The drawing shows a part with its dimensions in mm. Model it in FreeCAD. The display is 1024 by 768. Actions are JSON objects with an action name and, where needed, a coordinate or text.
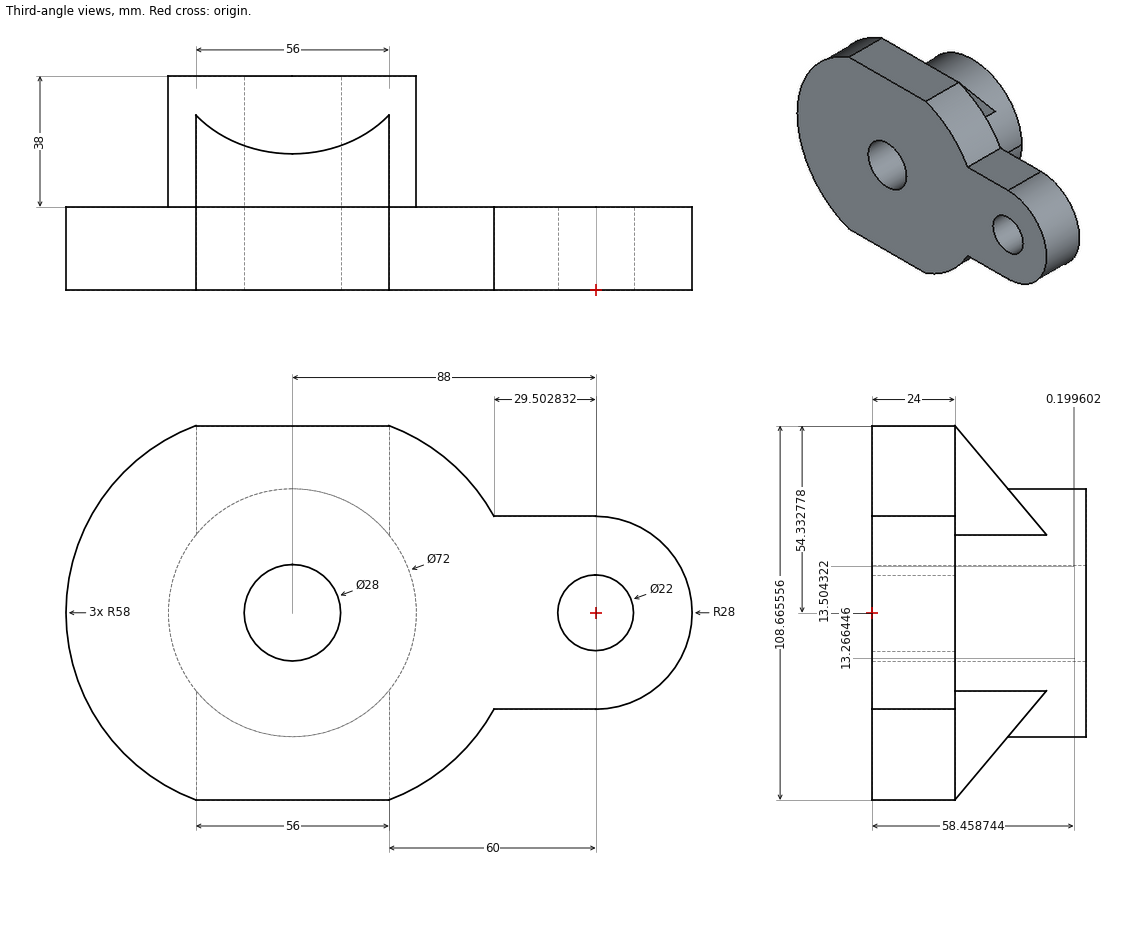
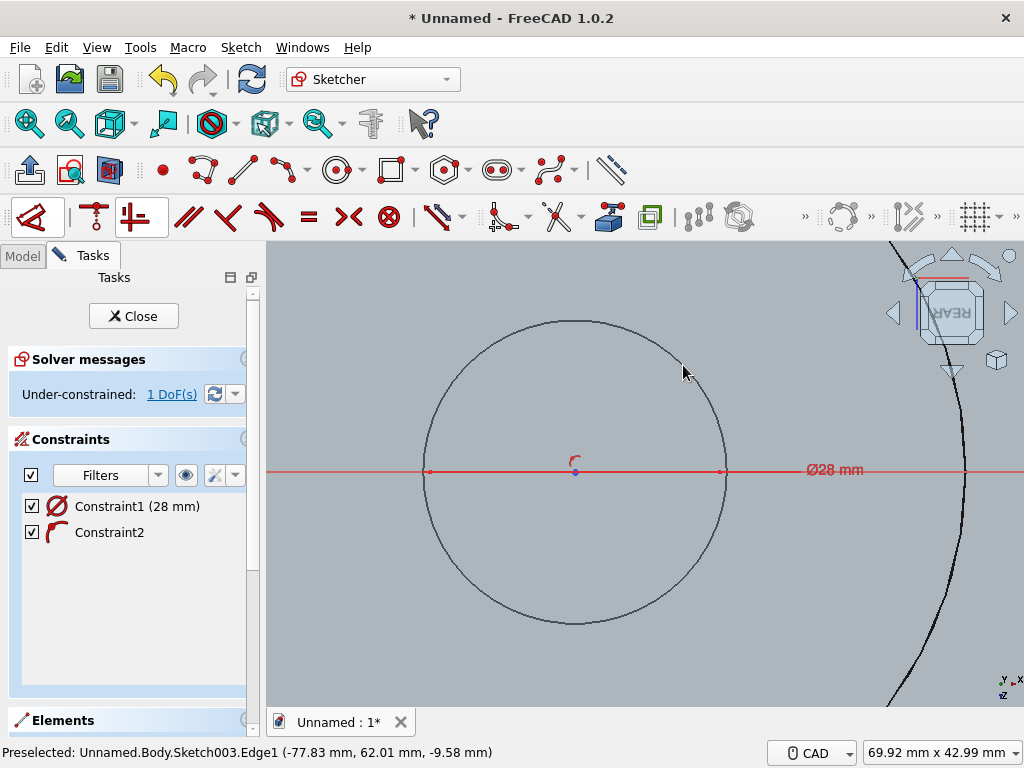
{"action": "left_click", "coordinate": [575, 472]}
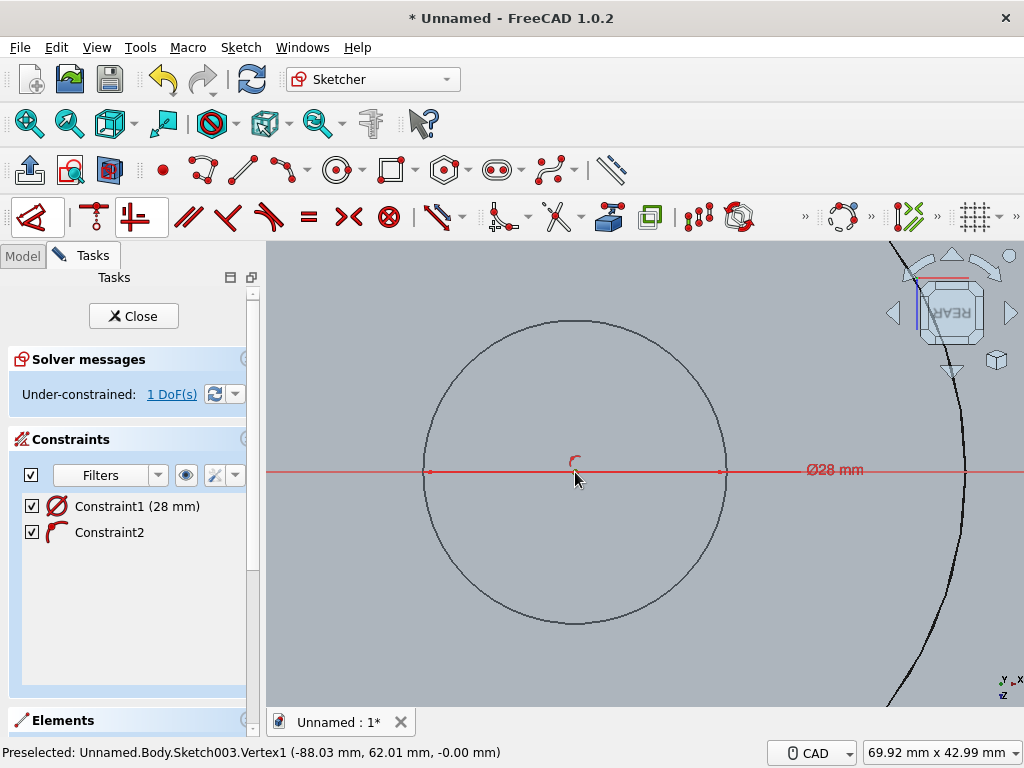
{"action": "key", "text": "l"}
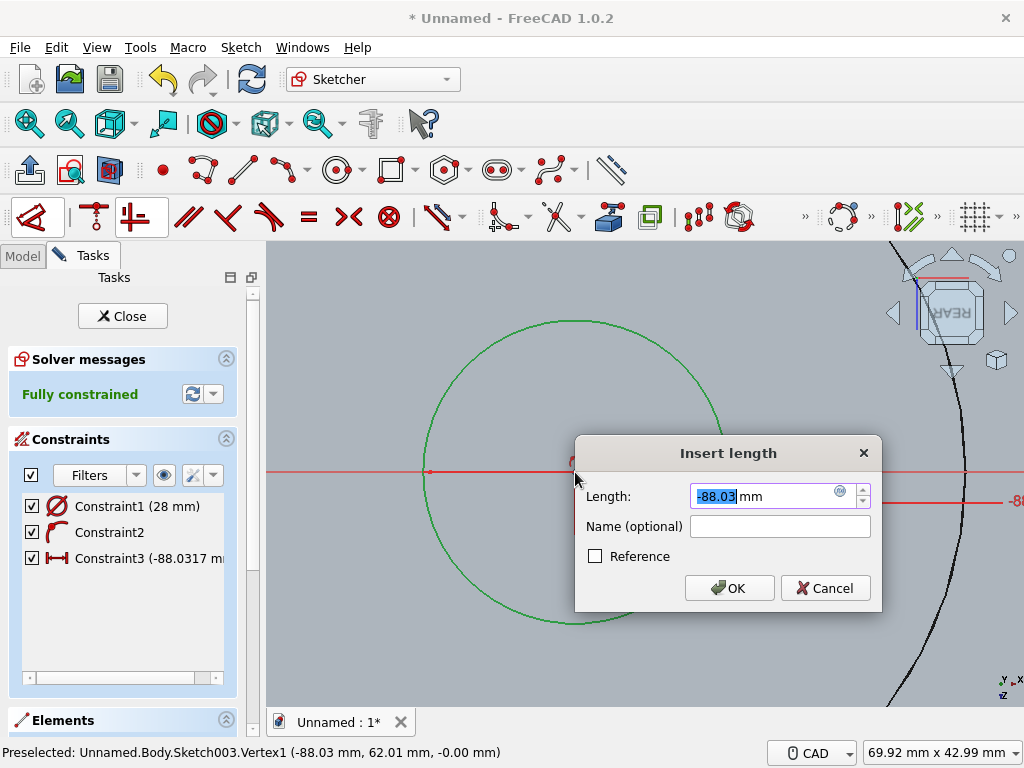
{"action": "type", "text": "-88"}
{"action": "key", "text": "Return"}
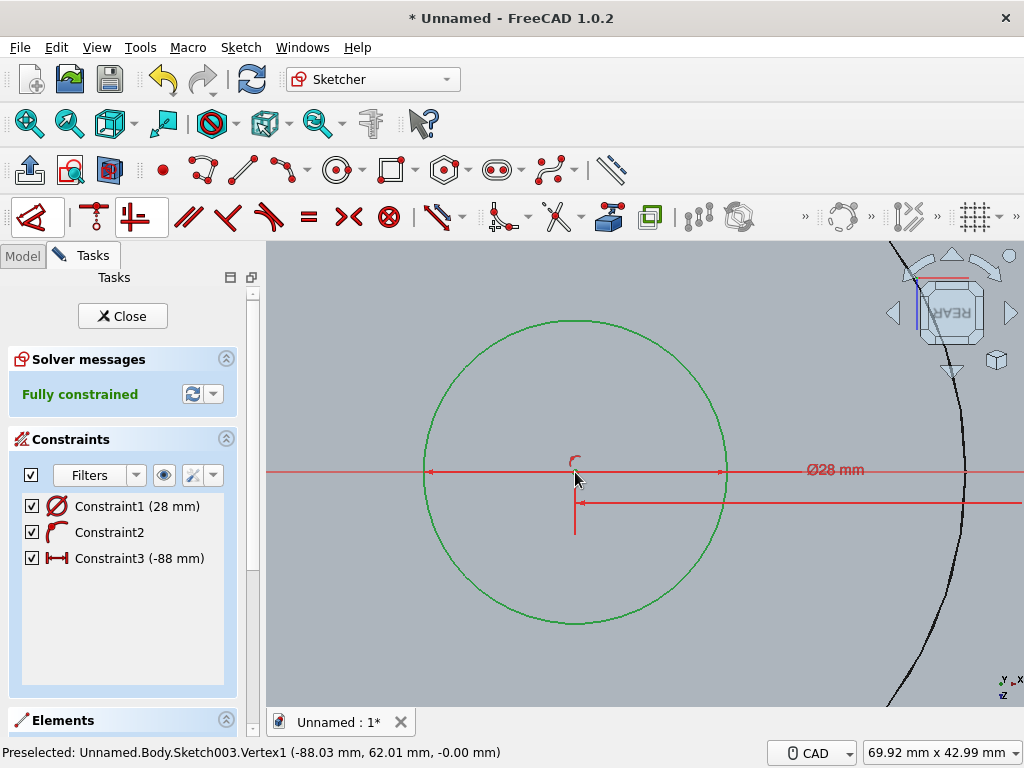
{"action": "left_click", "coordinate": [123, 316]}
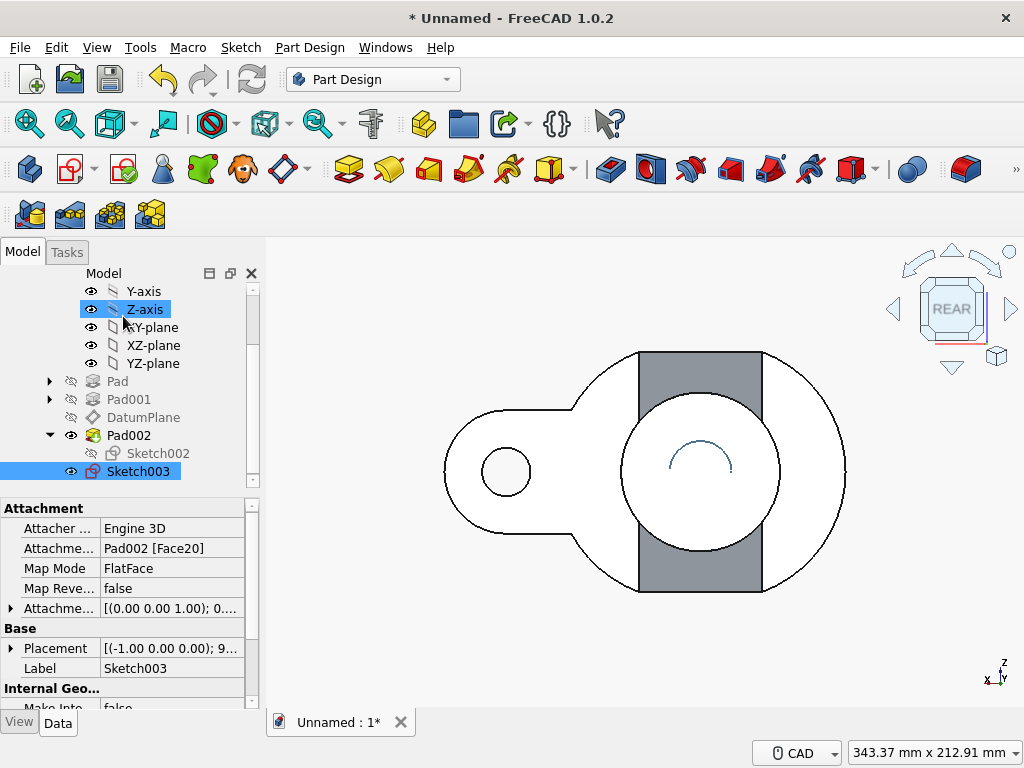
{"action": "left_click", "coordinate": [612, 170]}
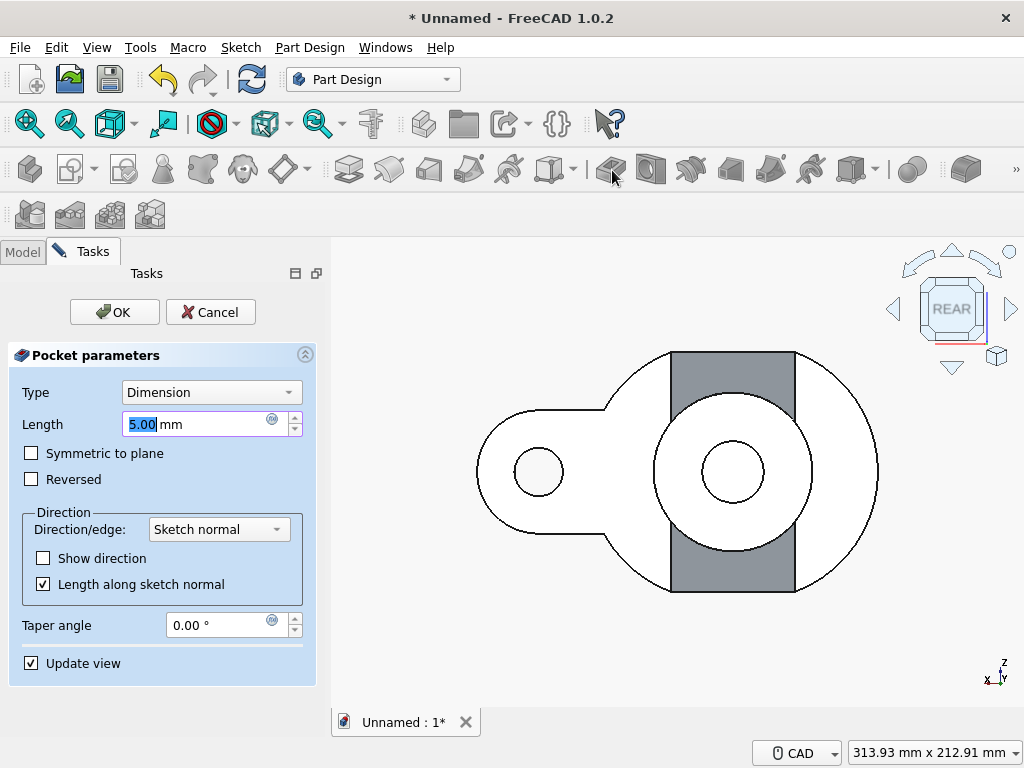
{"action": "left_click", "coordinate": [212, 392]}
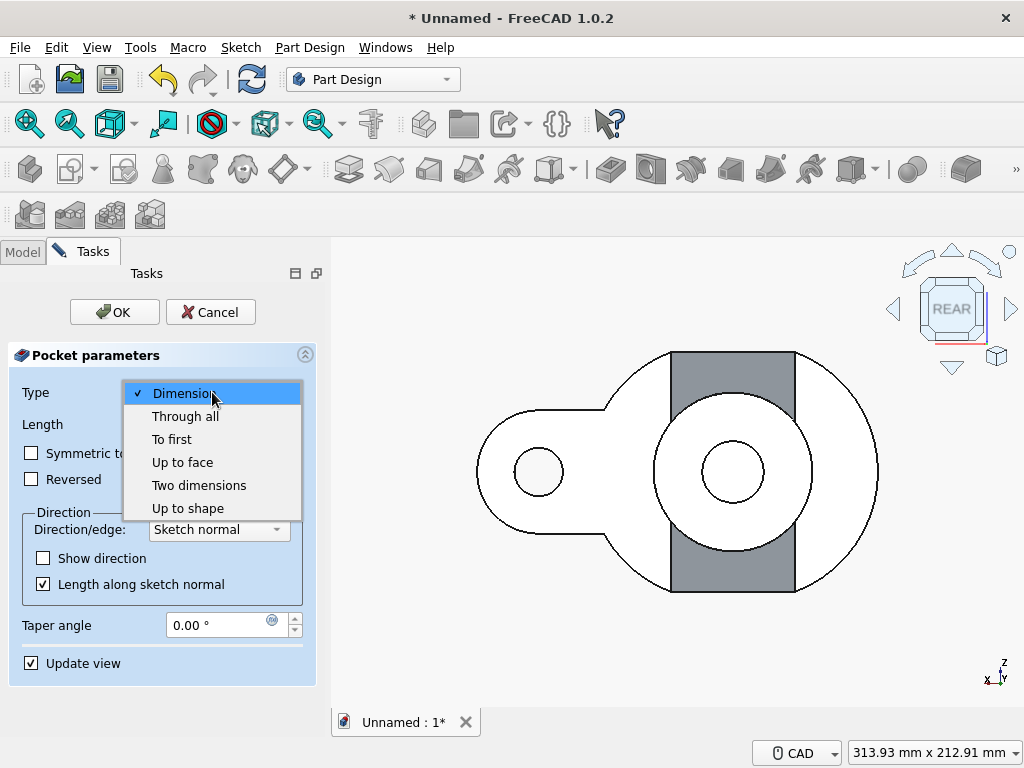
{"action": "left_click", "coordinate": [212, 440]}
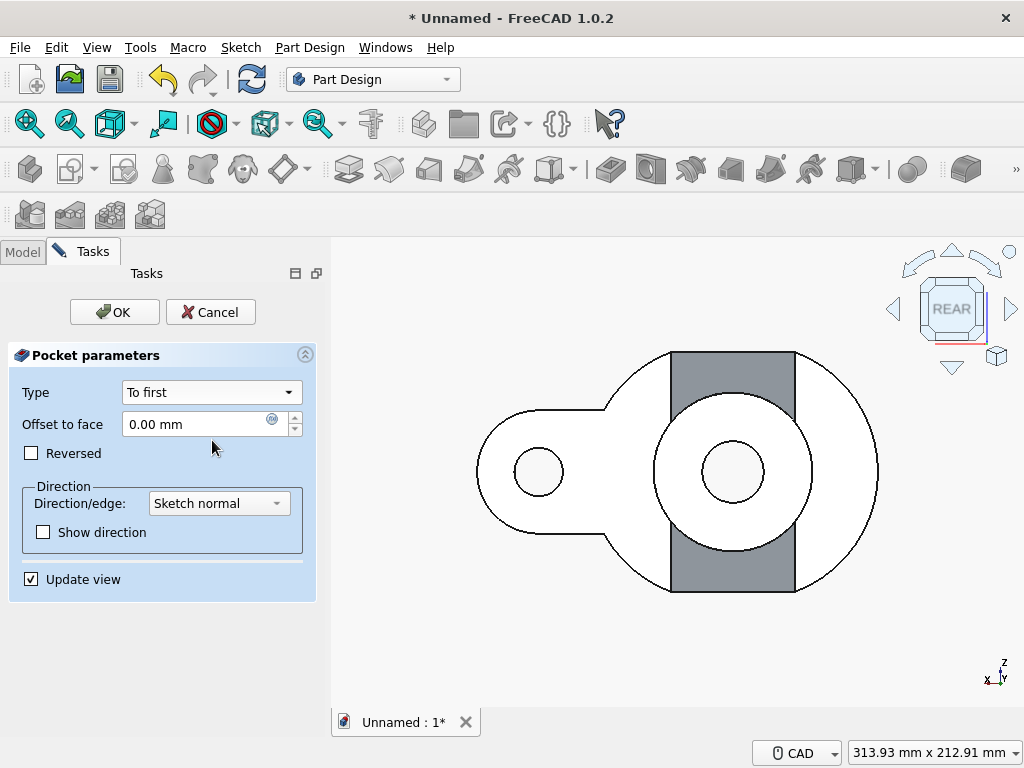
{"action": "left_click", "coordinate": [115, 312]}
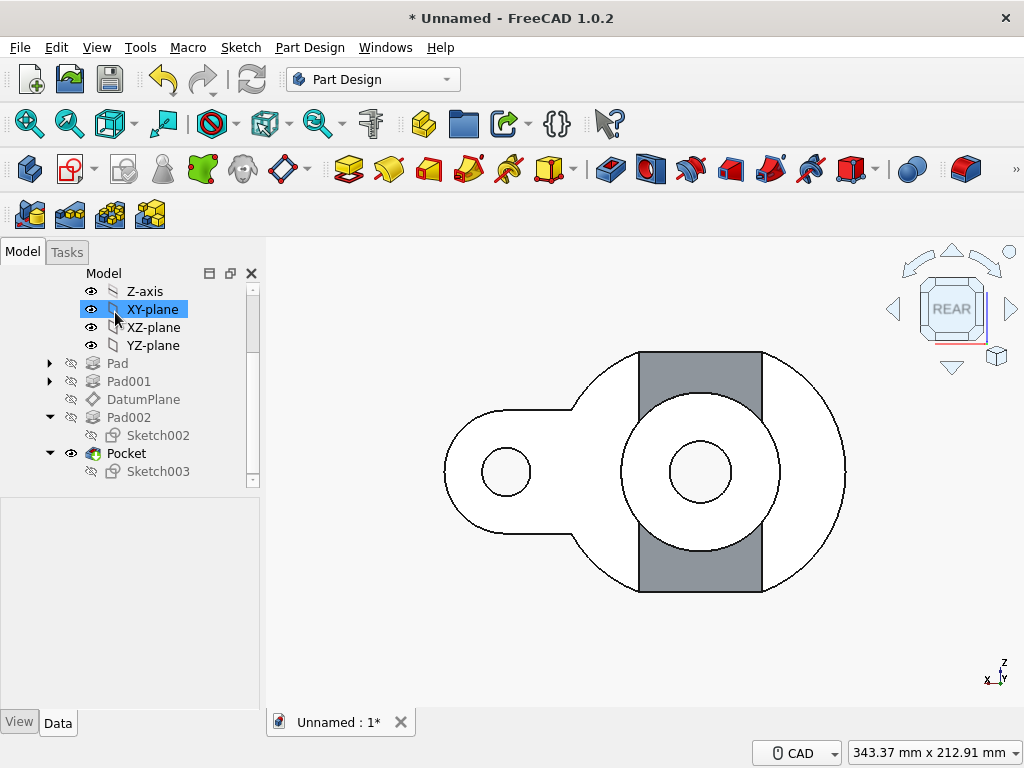
{"action": "key", "text": "0"}